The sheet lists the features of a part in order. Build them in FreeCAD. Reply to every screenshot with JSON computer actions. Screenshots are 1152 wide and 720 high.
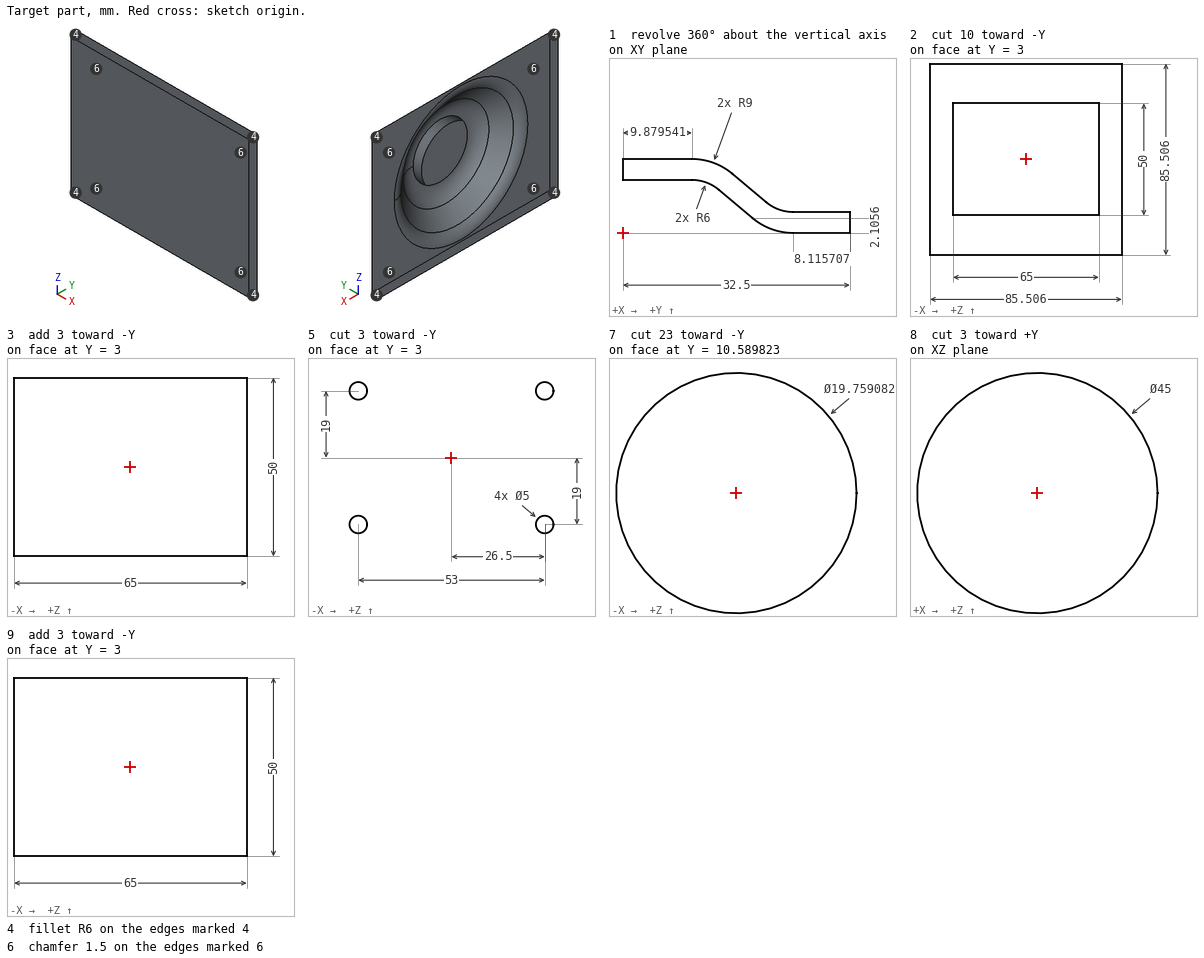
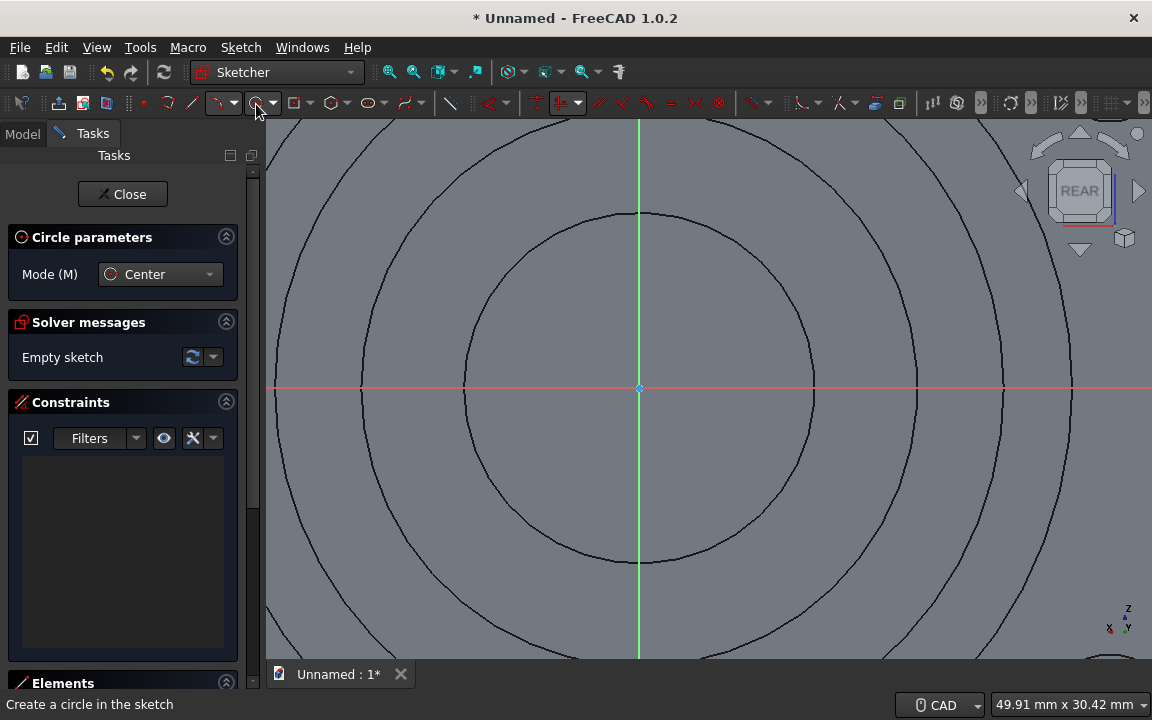
{"action": "left_click", "coordinate": [639, 388]}
{"action": "left_click", "coordinate": [763, 264]}
{"action": "key", "text": "Escape"}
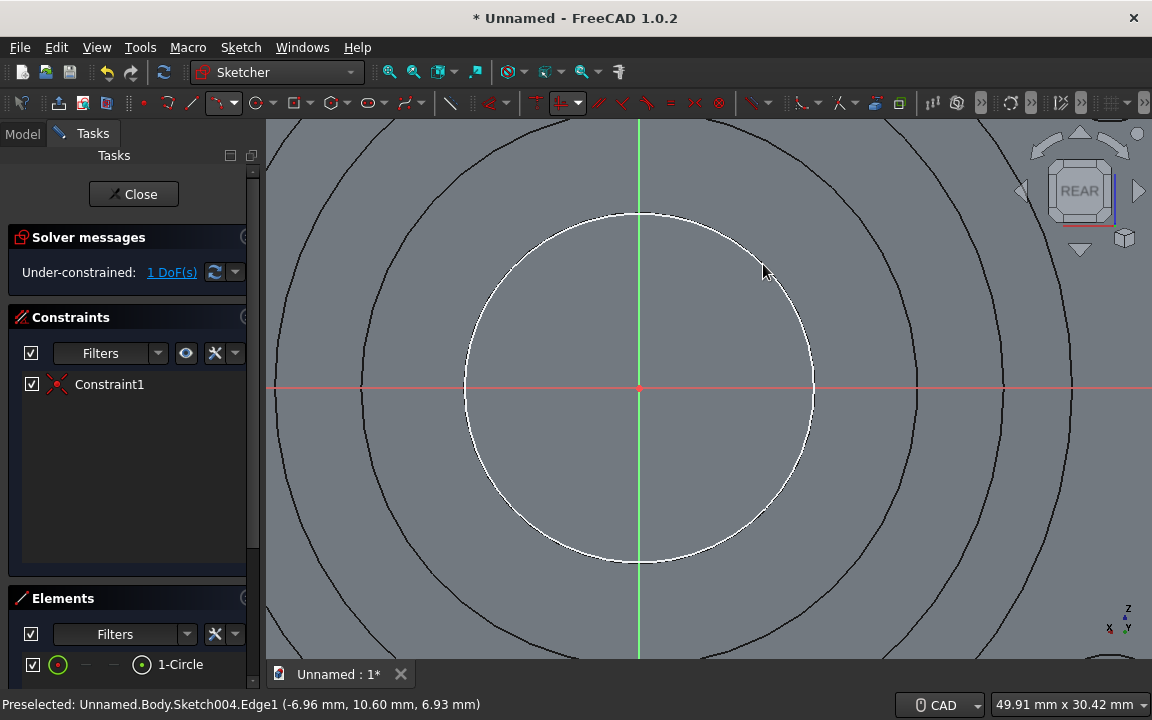
{"action": "left_click", "coordinate": [490, 104]}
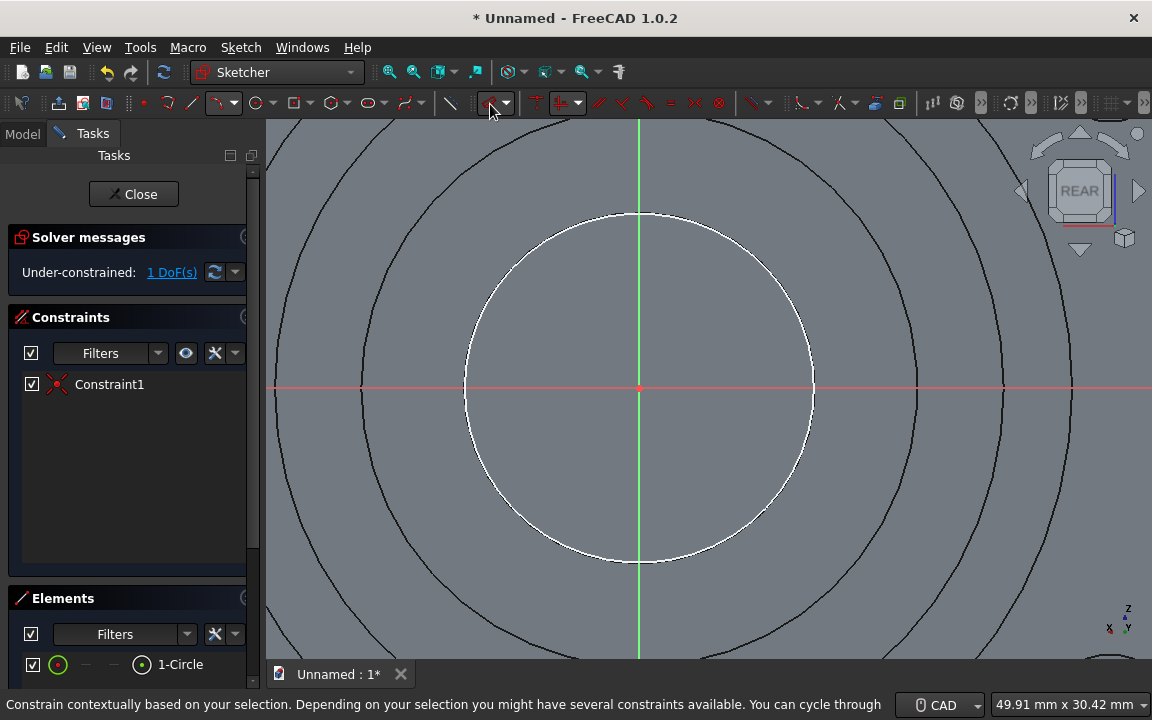
{"action": "left_click", "coordinate": [762, 264]}
{"action": "left_click", "coordinate": [784, 241]}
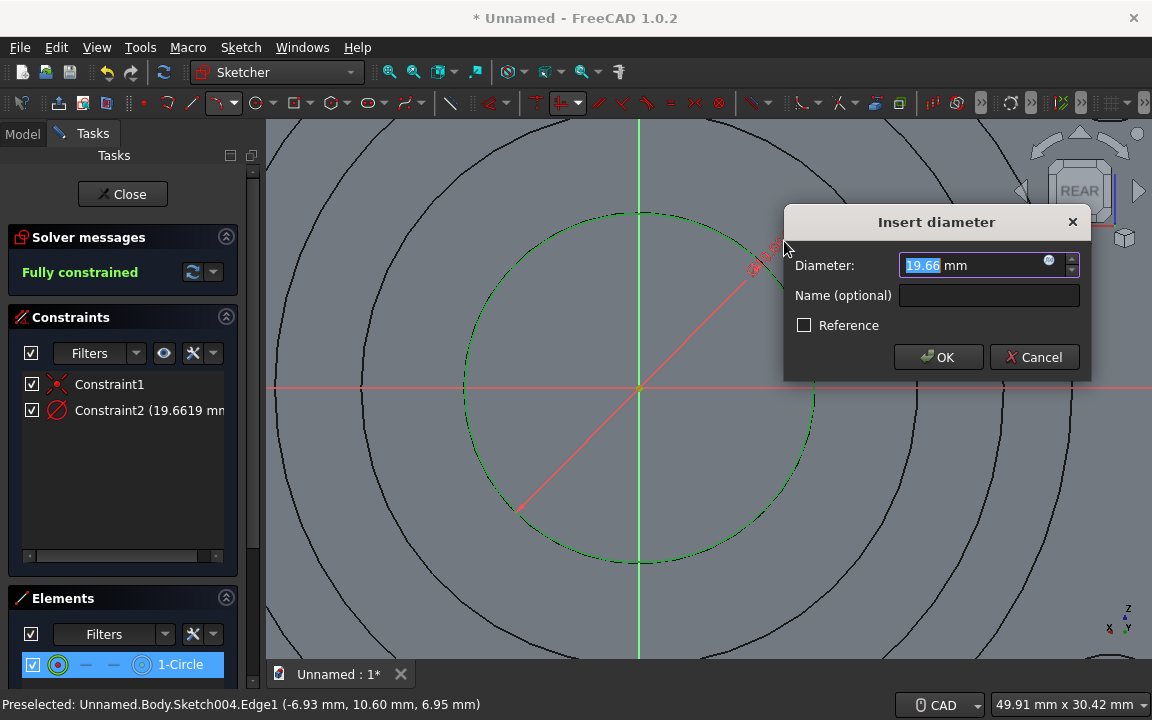
{"action": "type", "text": "19.759082"}
{"action": "key", "text": "Return"}
{"action": "key", "text": "Escape"}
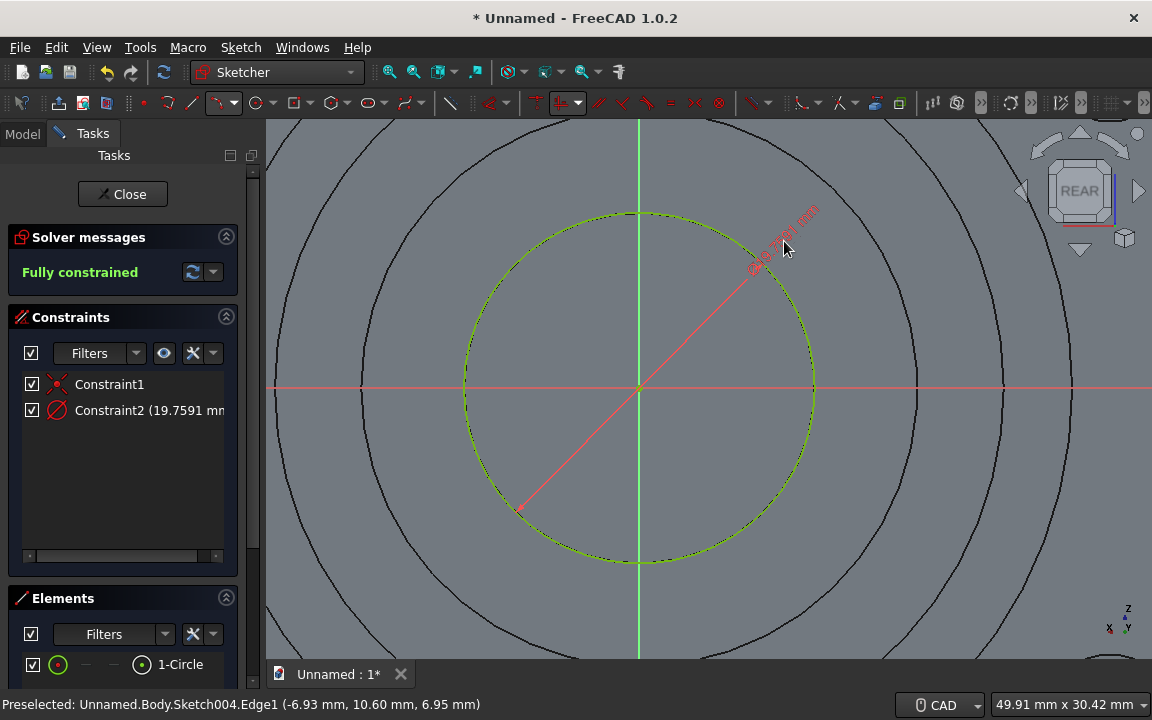
{"action": "left_click", "coordinate": [123, 194]}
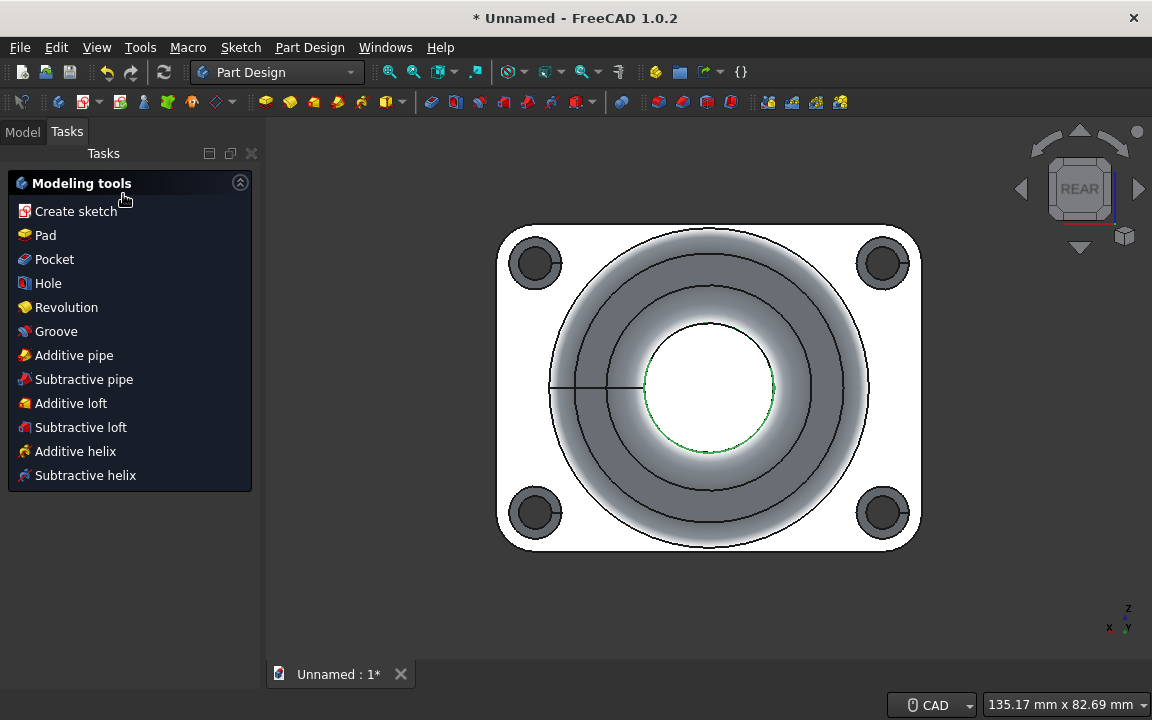
{"action": "left_click", "coordinate": [432, 102]}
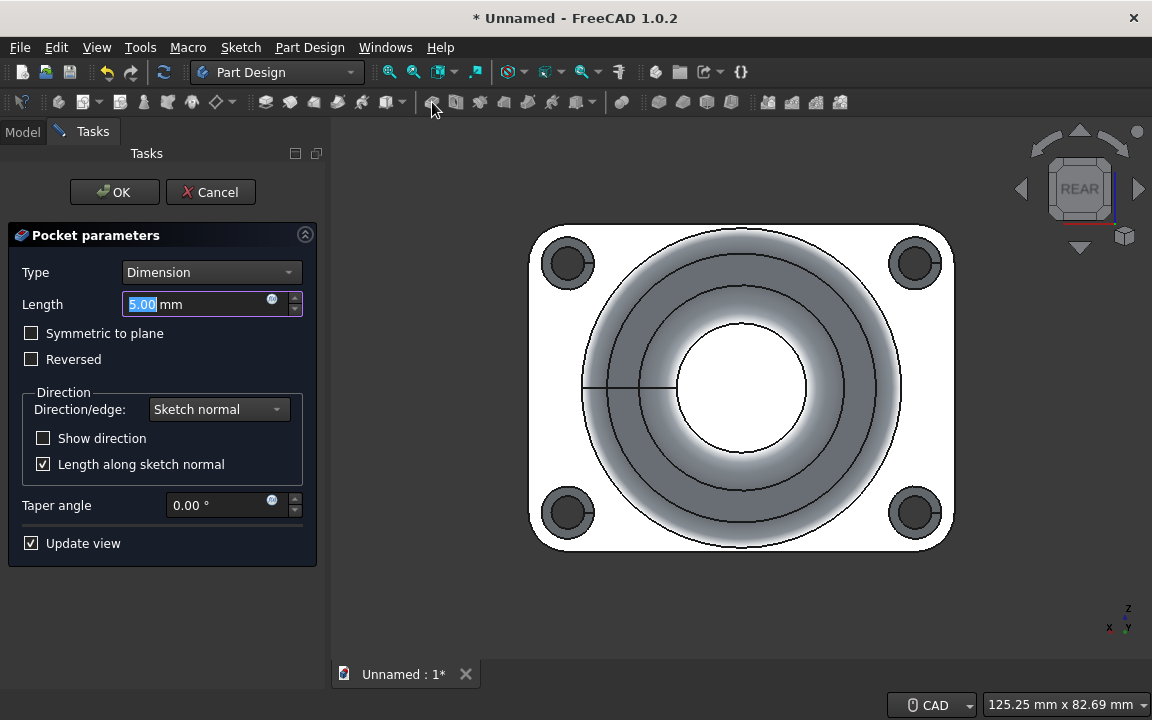
{"action": "type", "text": "23"}
{"action": "key", "text": "Tab"}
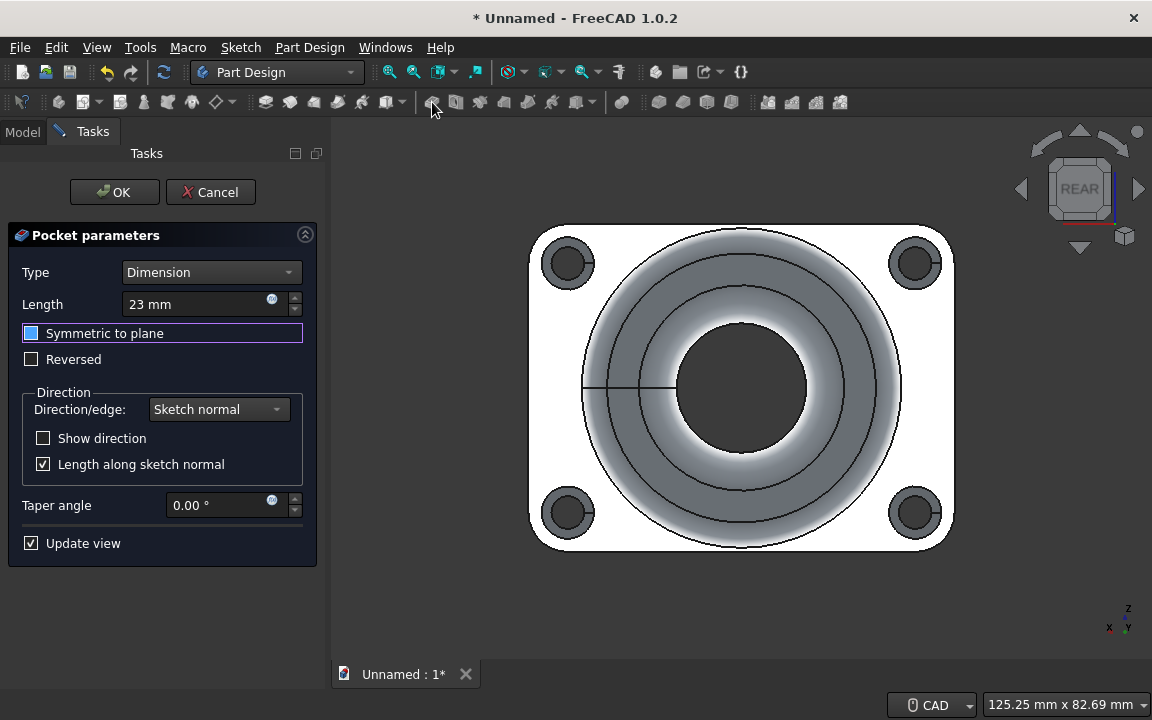
{"action": "left_click", "coordinate": [115, 192]}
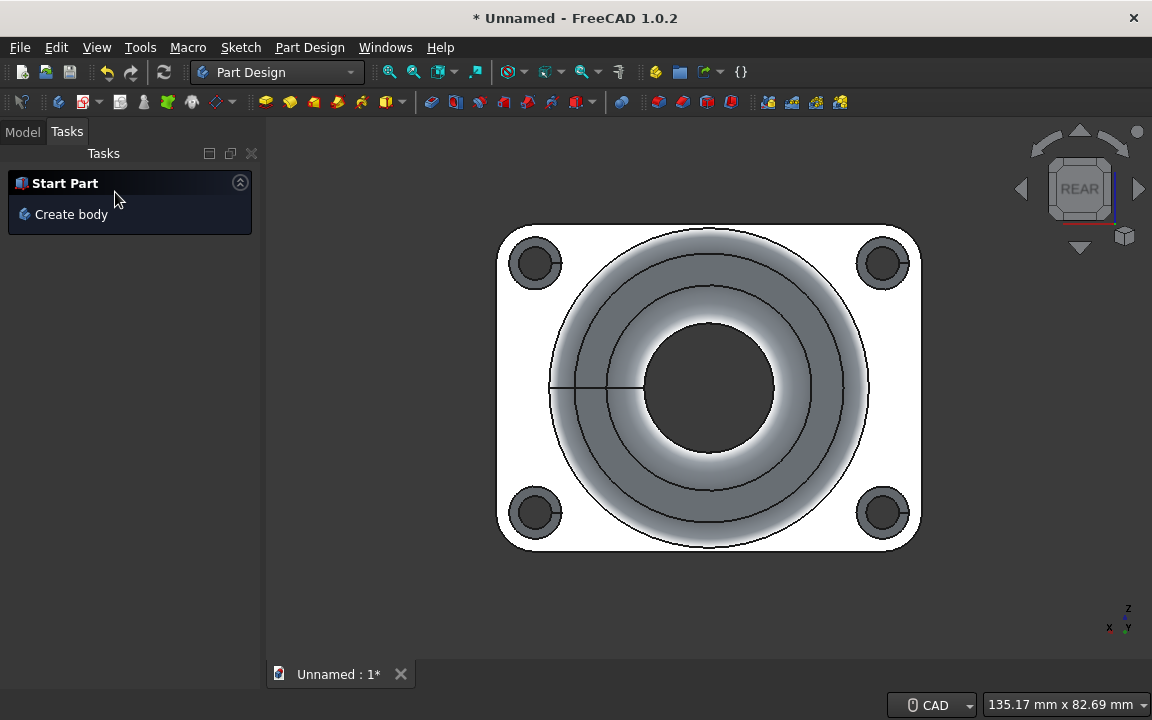
{"action": "left_click", "coordinate": [84, 102]}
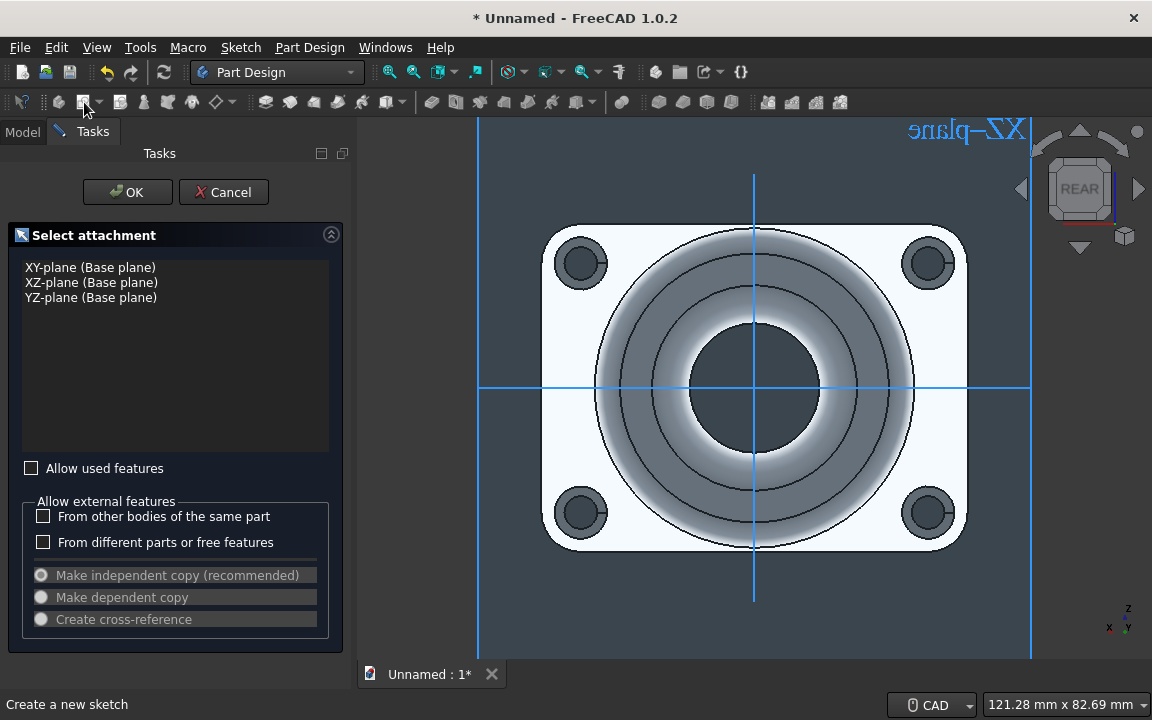
{"action": "left_click", "coordinate": [82, 282]}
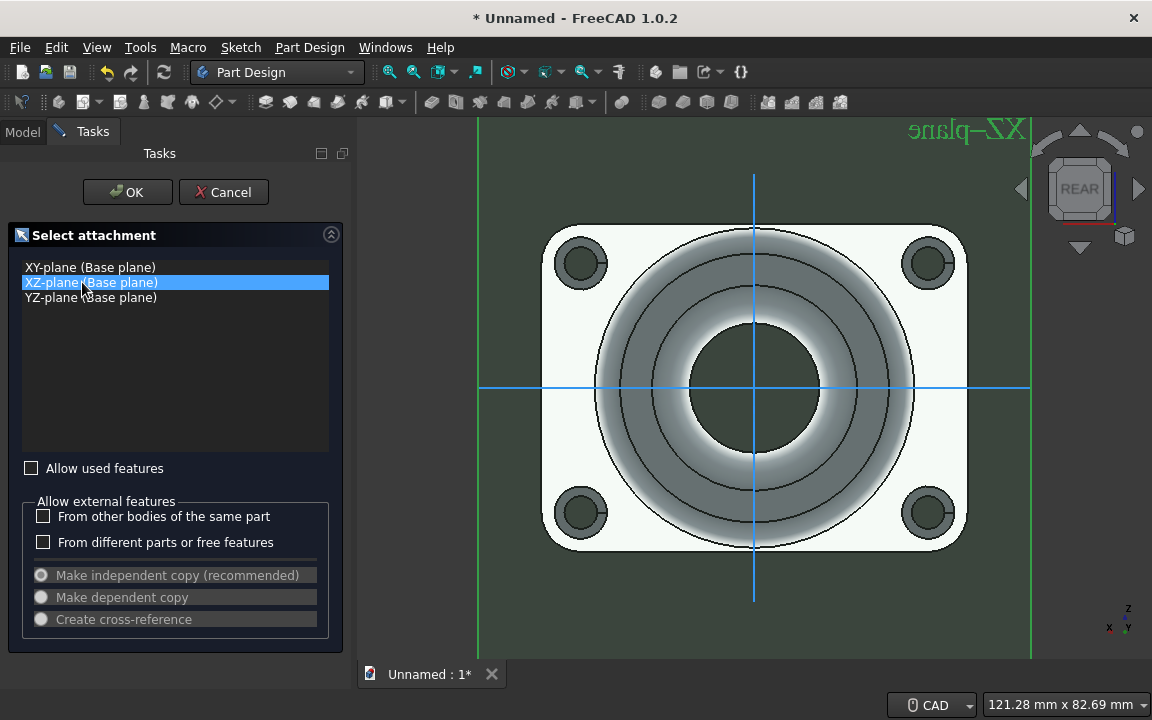
{"action": "left_click", "coordinate": [128, 192]}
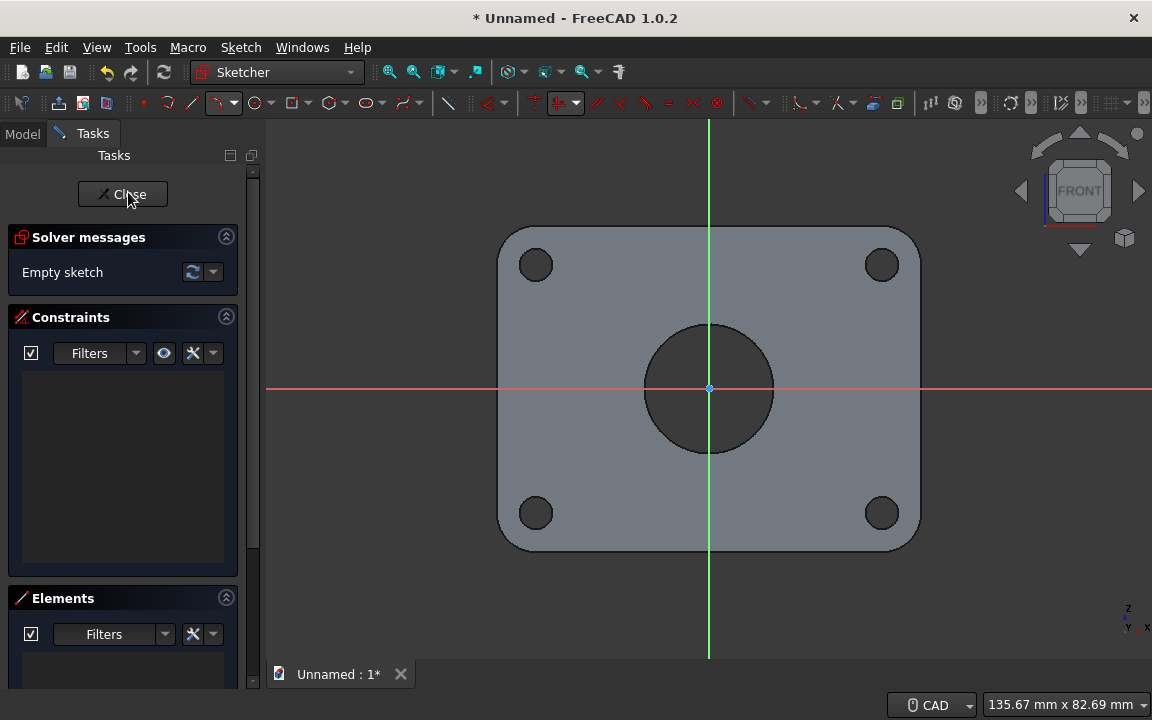
{"action": "left_click", "coordinate": [256, 104]}